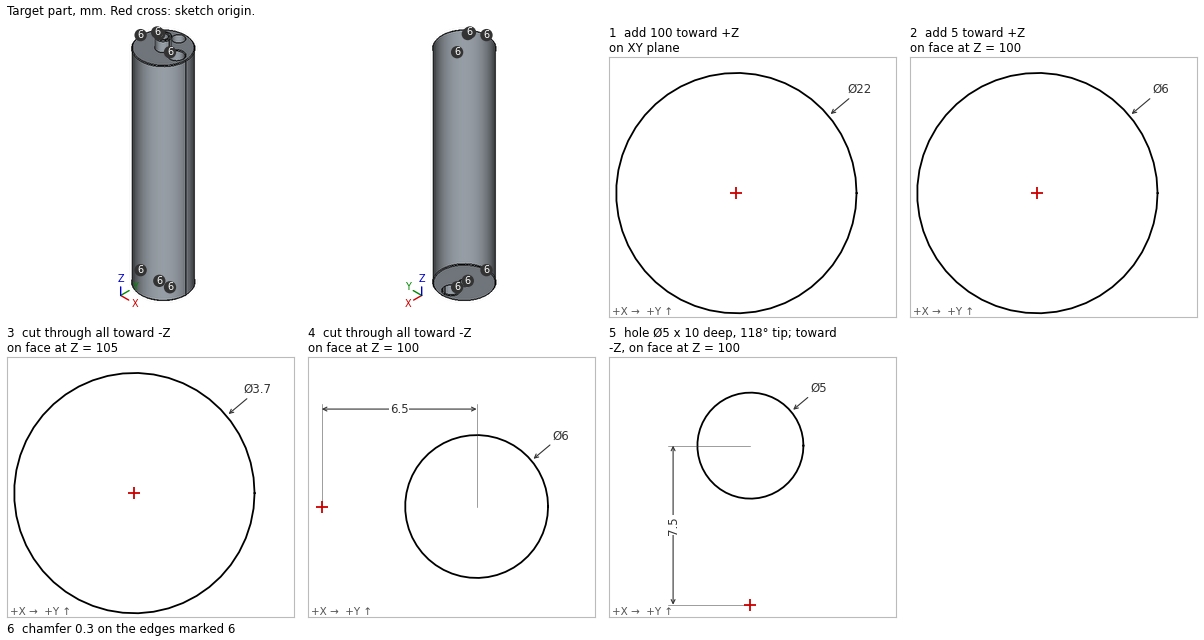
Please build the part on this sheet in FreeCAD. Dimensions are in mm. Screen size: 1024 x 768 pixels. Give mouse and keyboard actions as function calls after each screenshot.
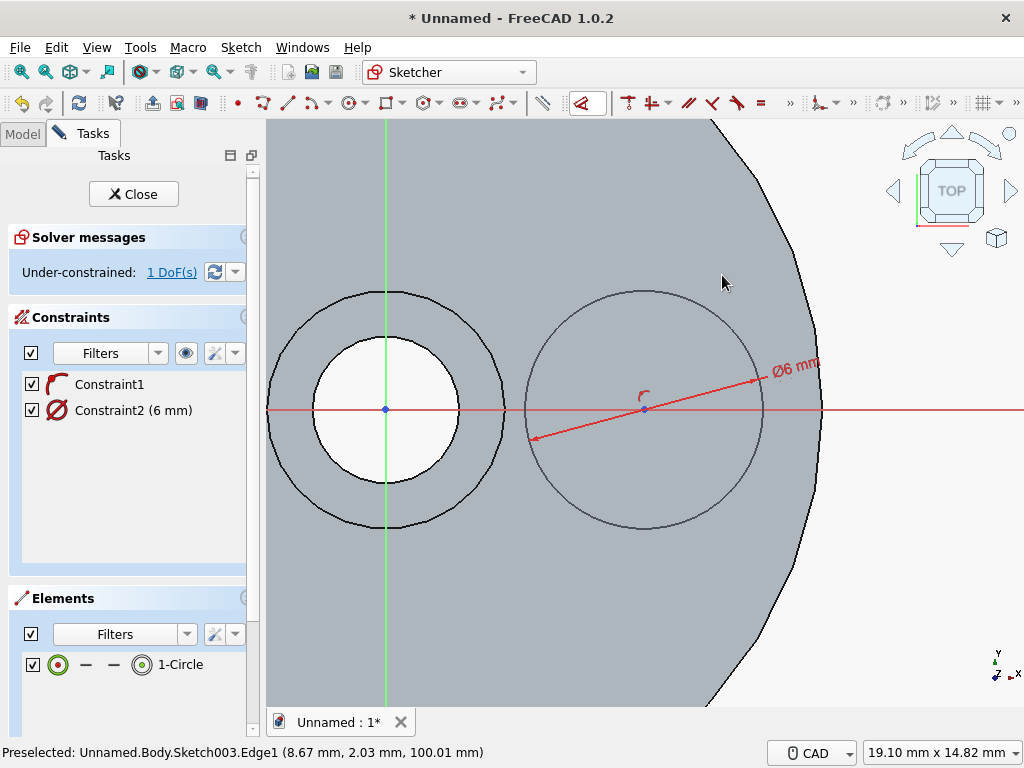
click(644, 410)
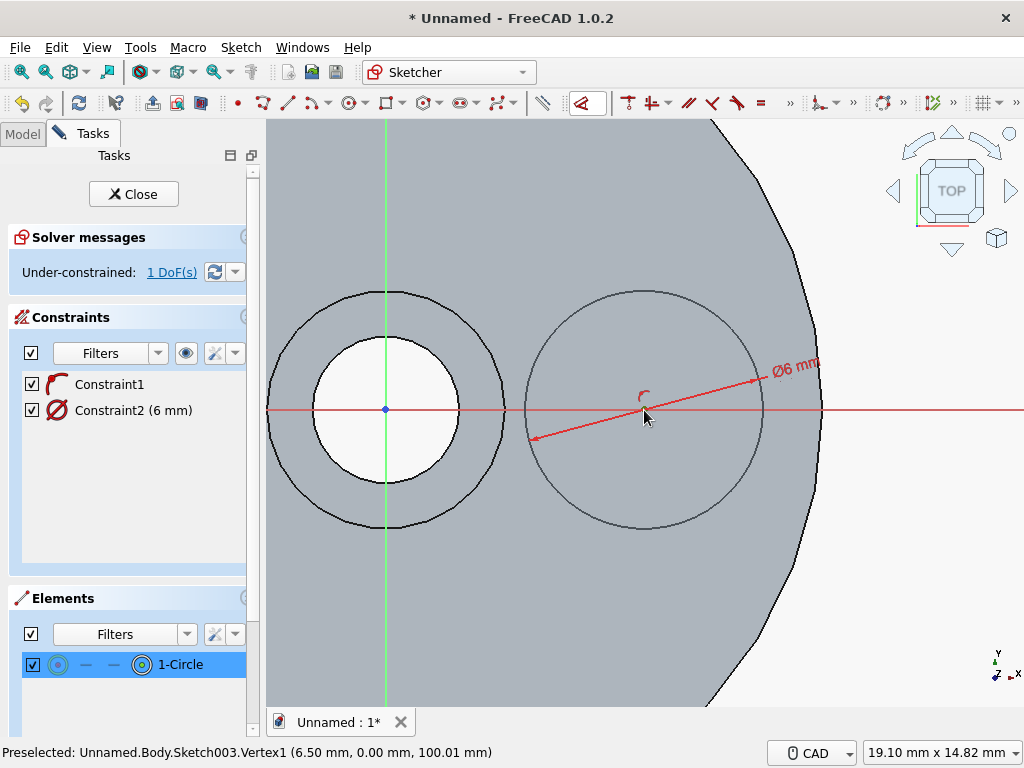
click(600, 104)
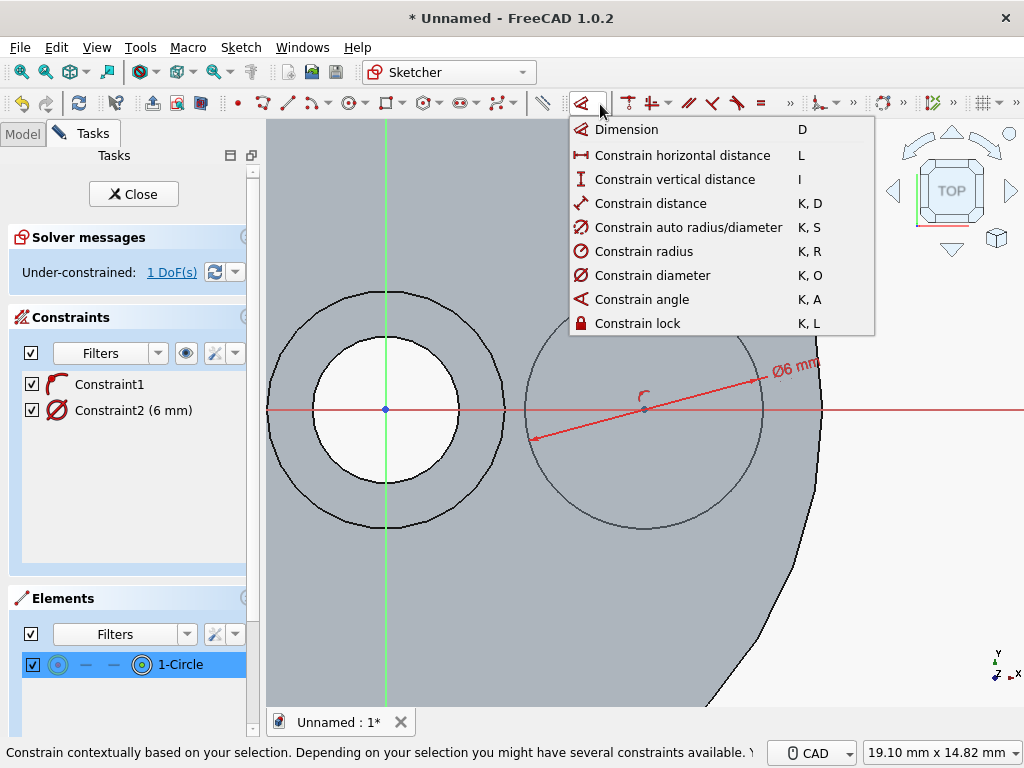
click(722, 155)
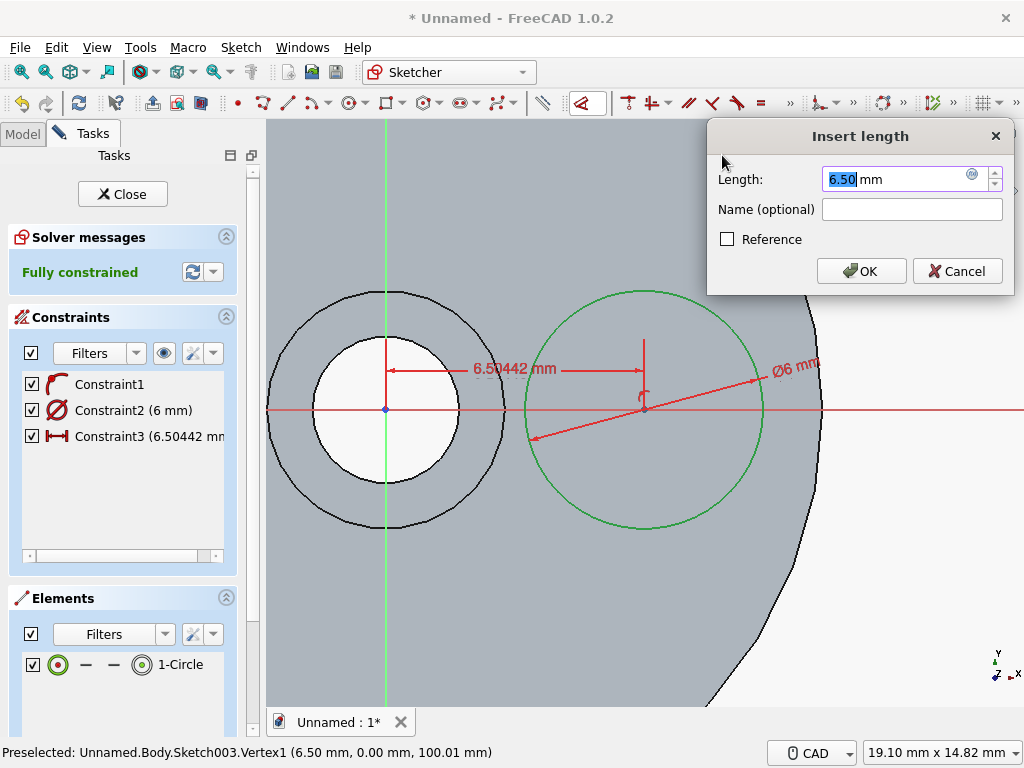
text(6.5)
key(Return)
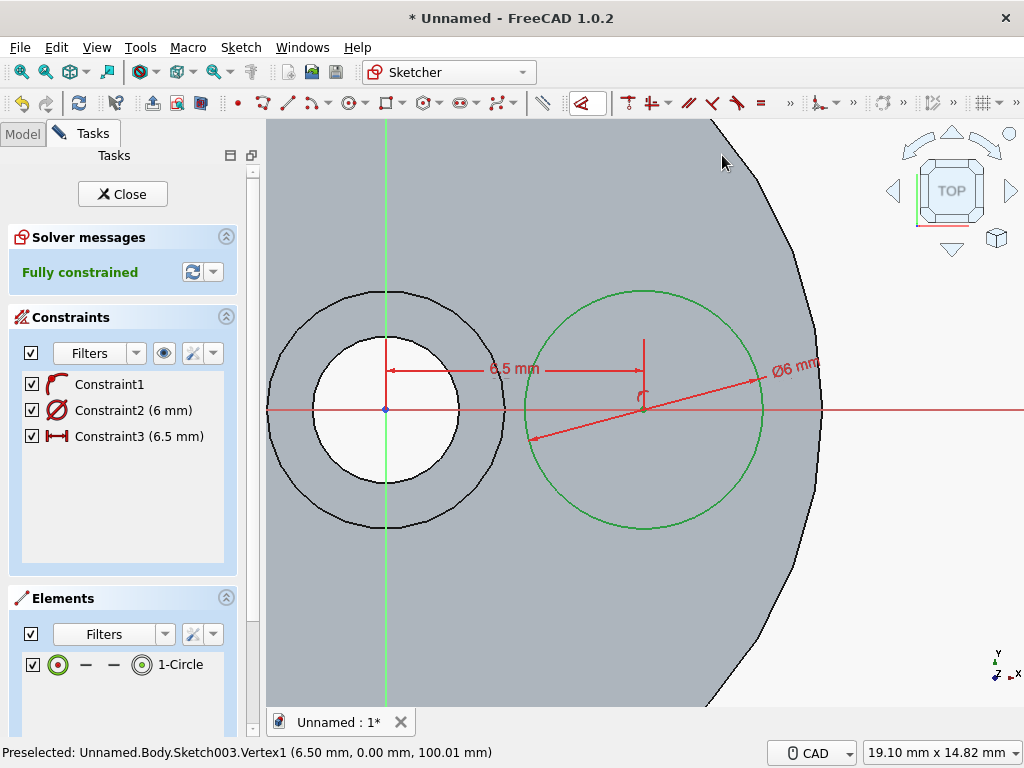
click(123, 194)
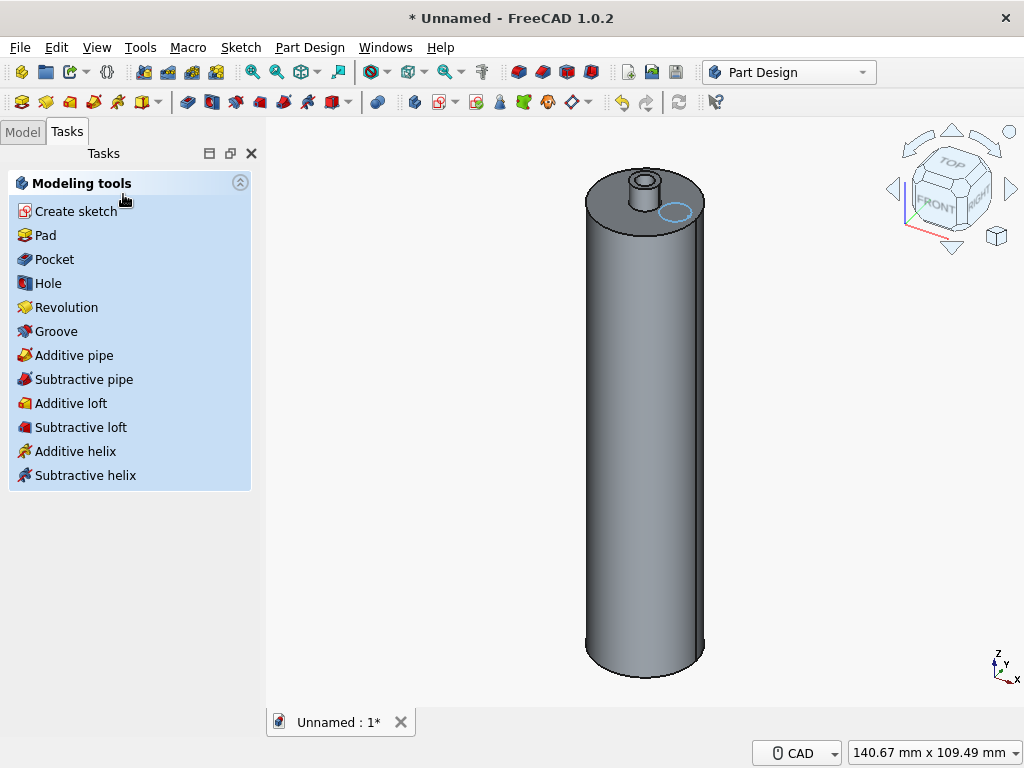
click(188, 102)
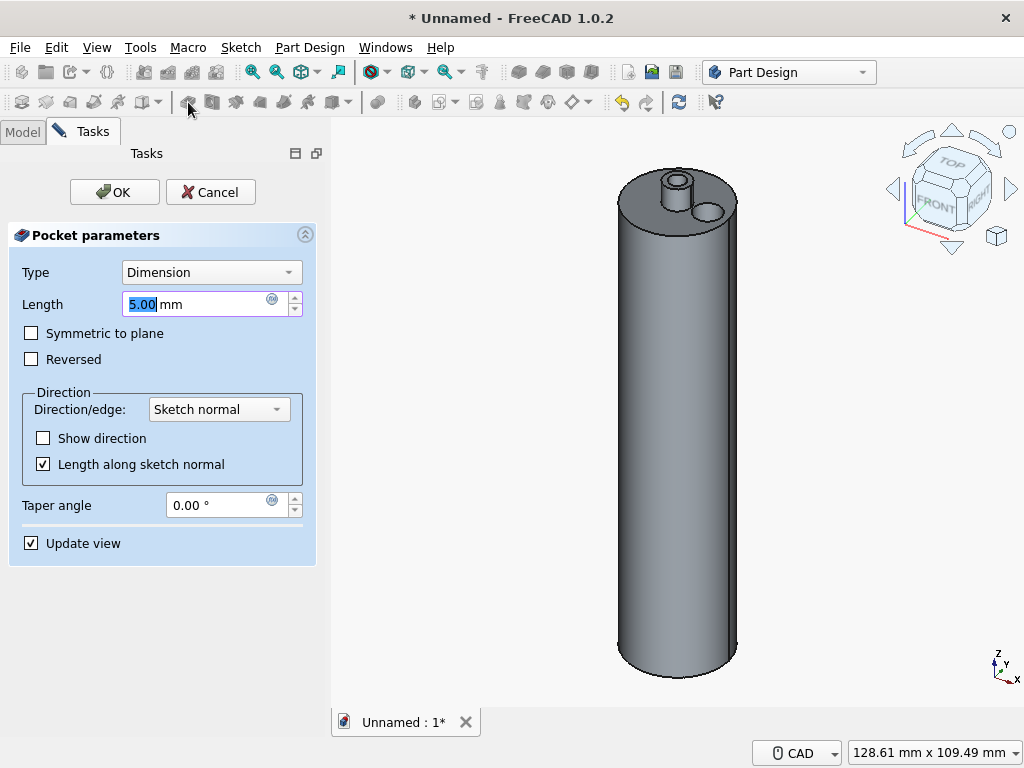
click(212, 272)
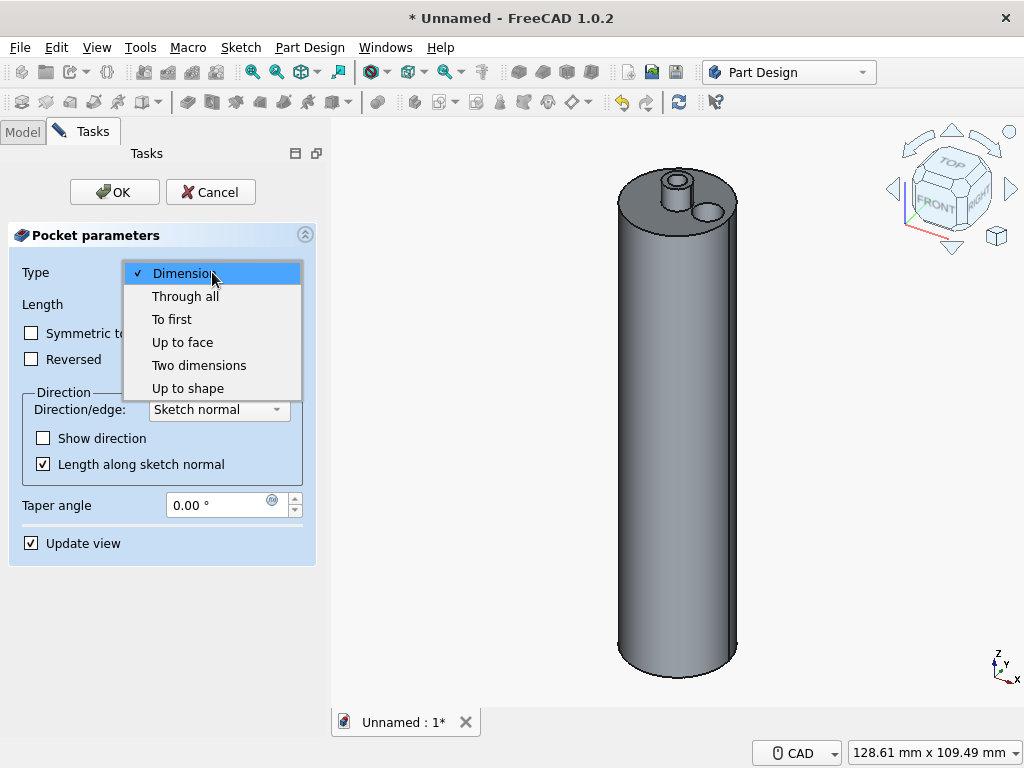
click(212, 296)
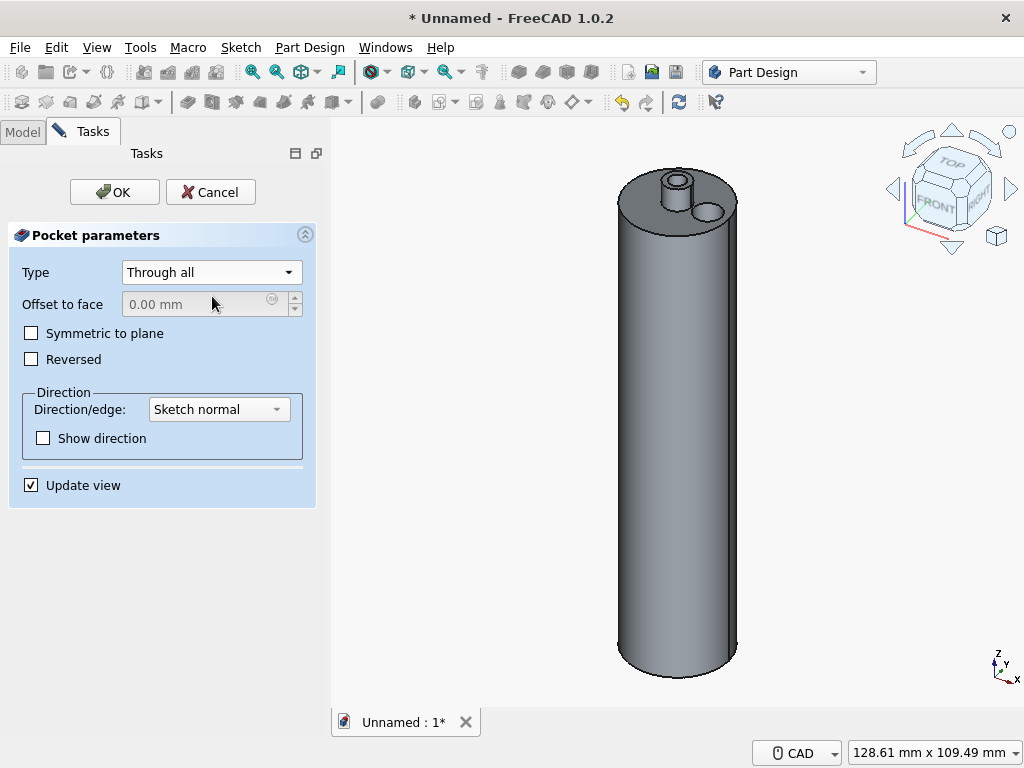
click(115, 192)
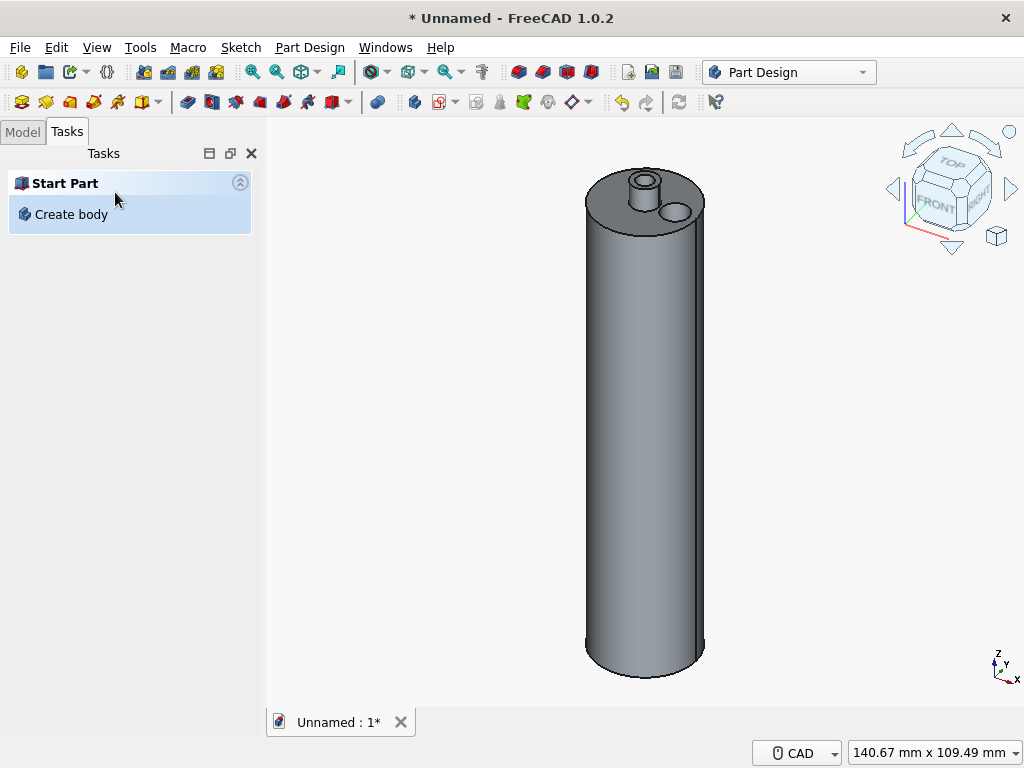
click(677, 189)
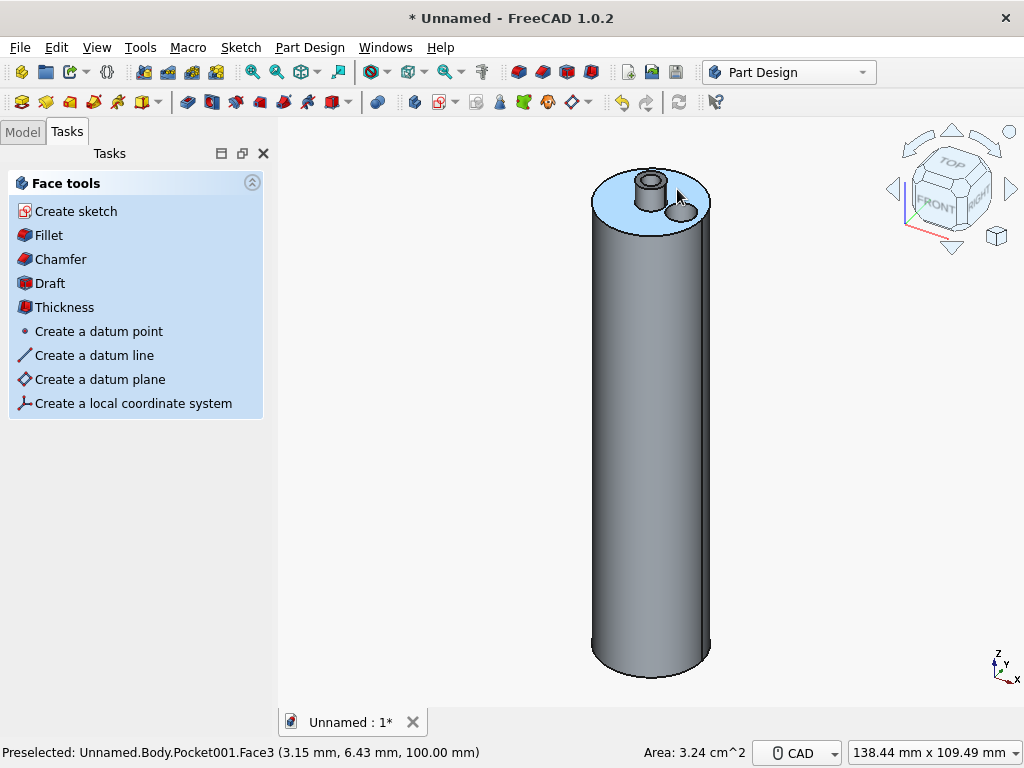
click(440, 102)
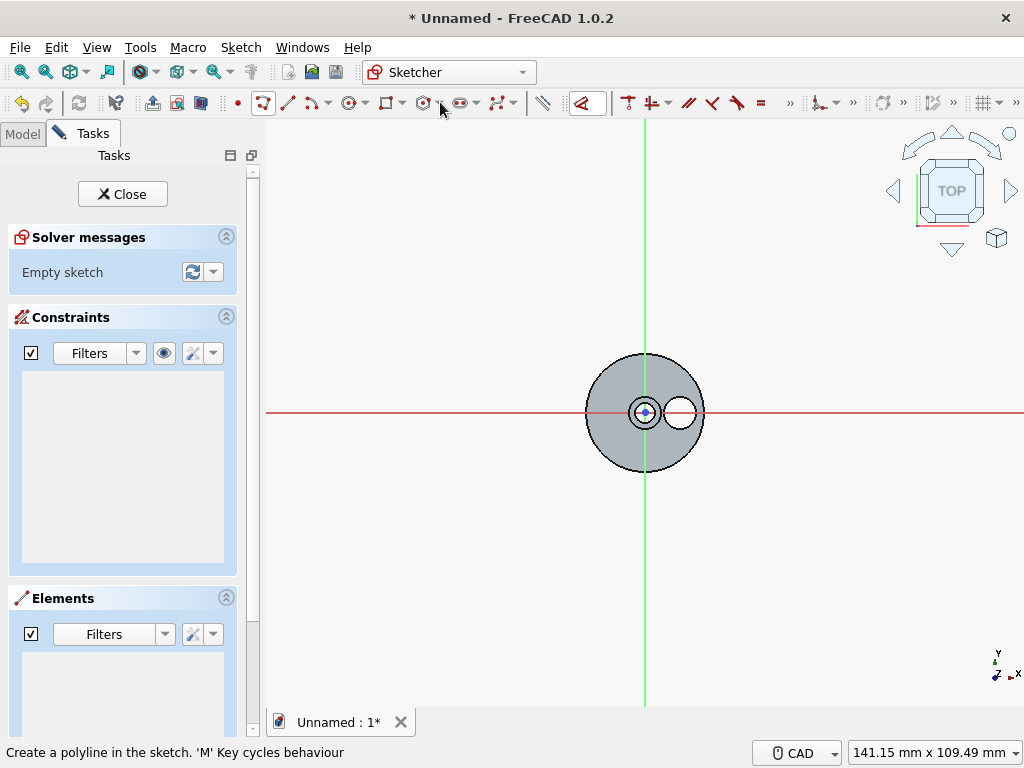
key(q)
key(s)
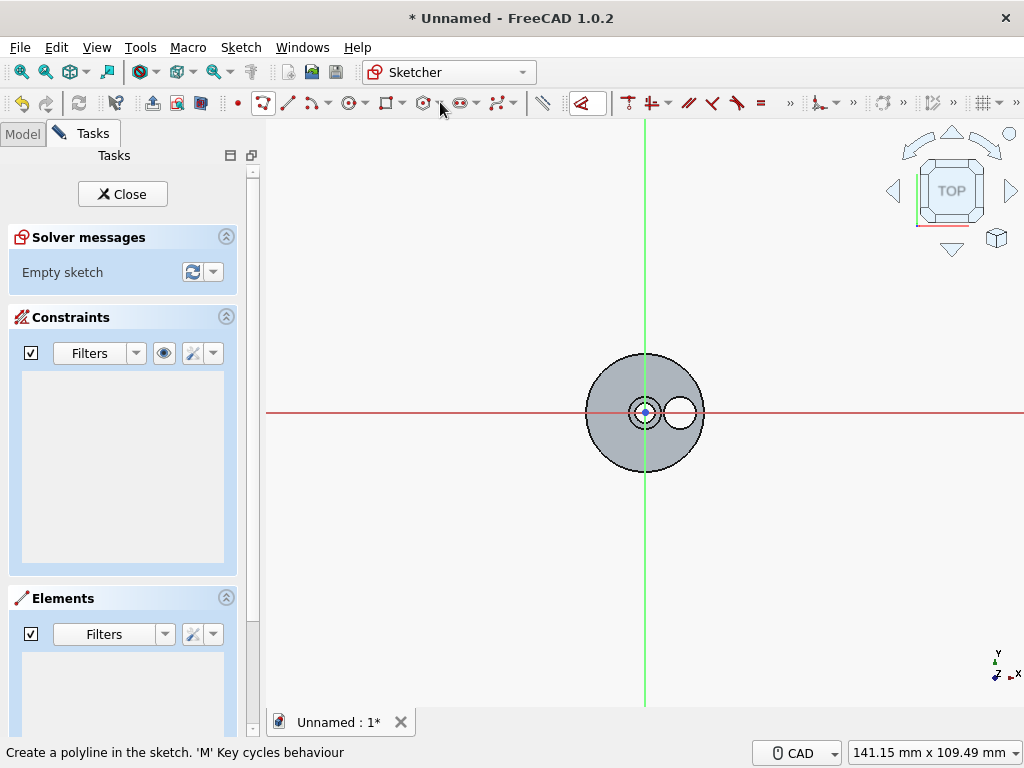
scroll(656, 382, up, 10)